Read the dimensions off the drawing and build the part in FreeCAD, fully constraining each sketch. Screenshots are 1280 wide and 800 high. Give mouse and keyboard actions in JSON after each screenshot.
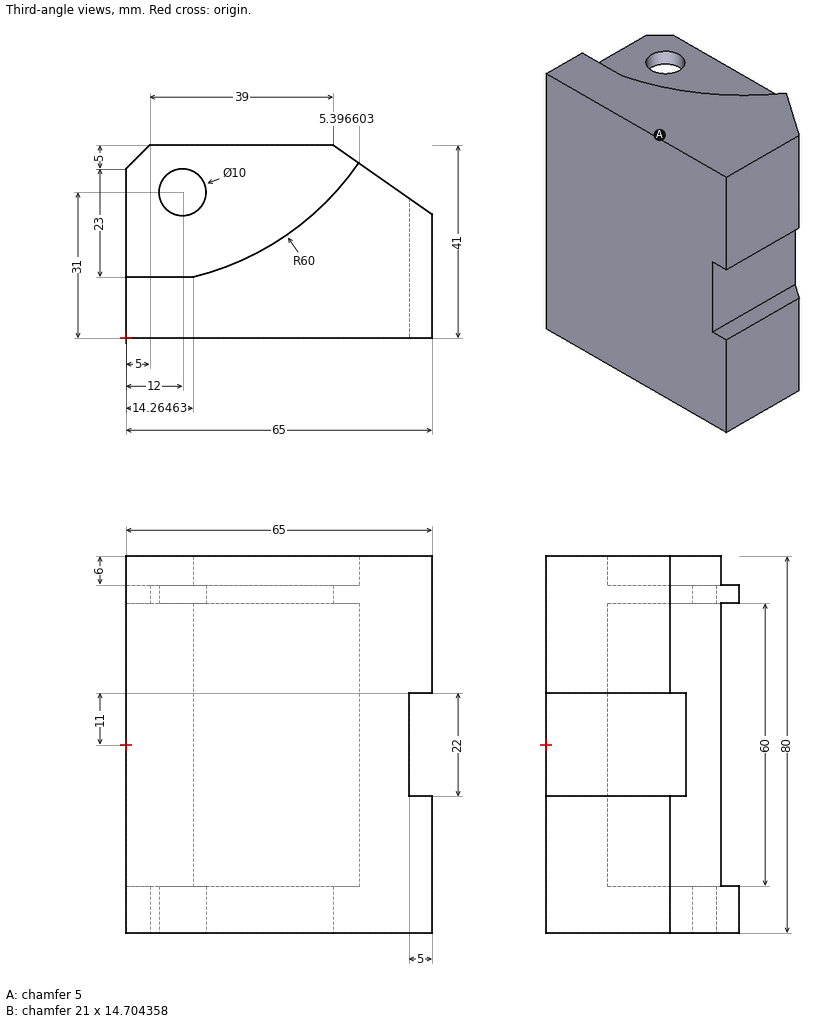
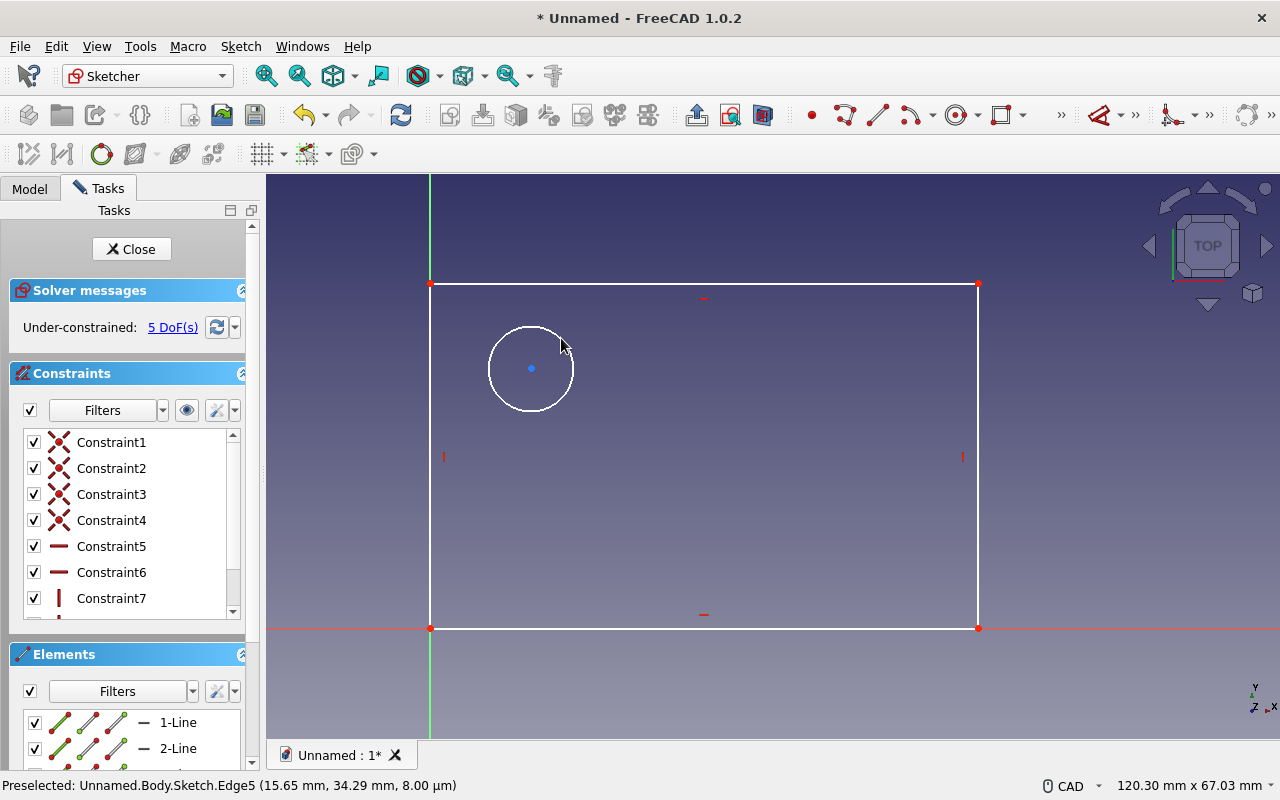
{"action": "key", "text": "d"}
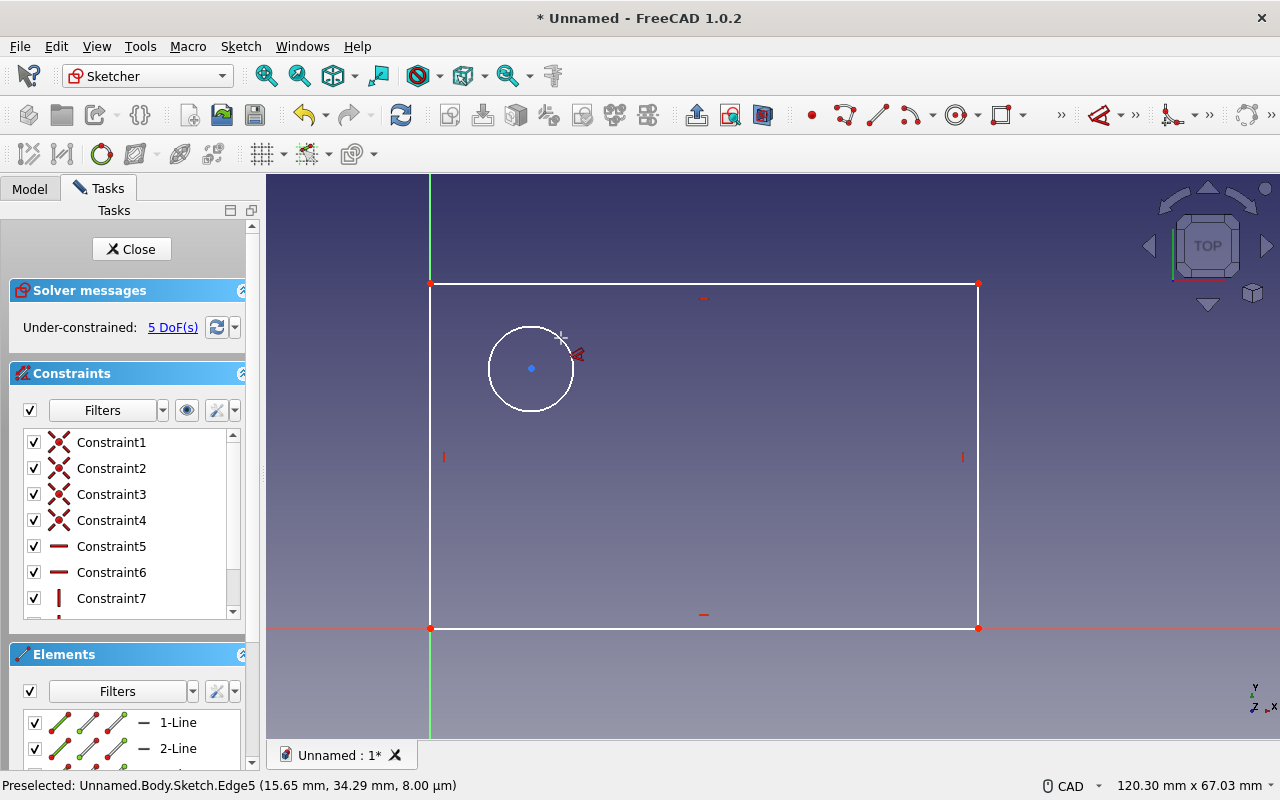
{"action": "left_click", "coordinate": [561, 339]}
{"action": "left_click", "coordinate": [584, 316]}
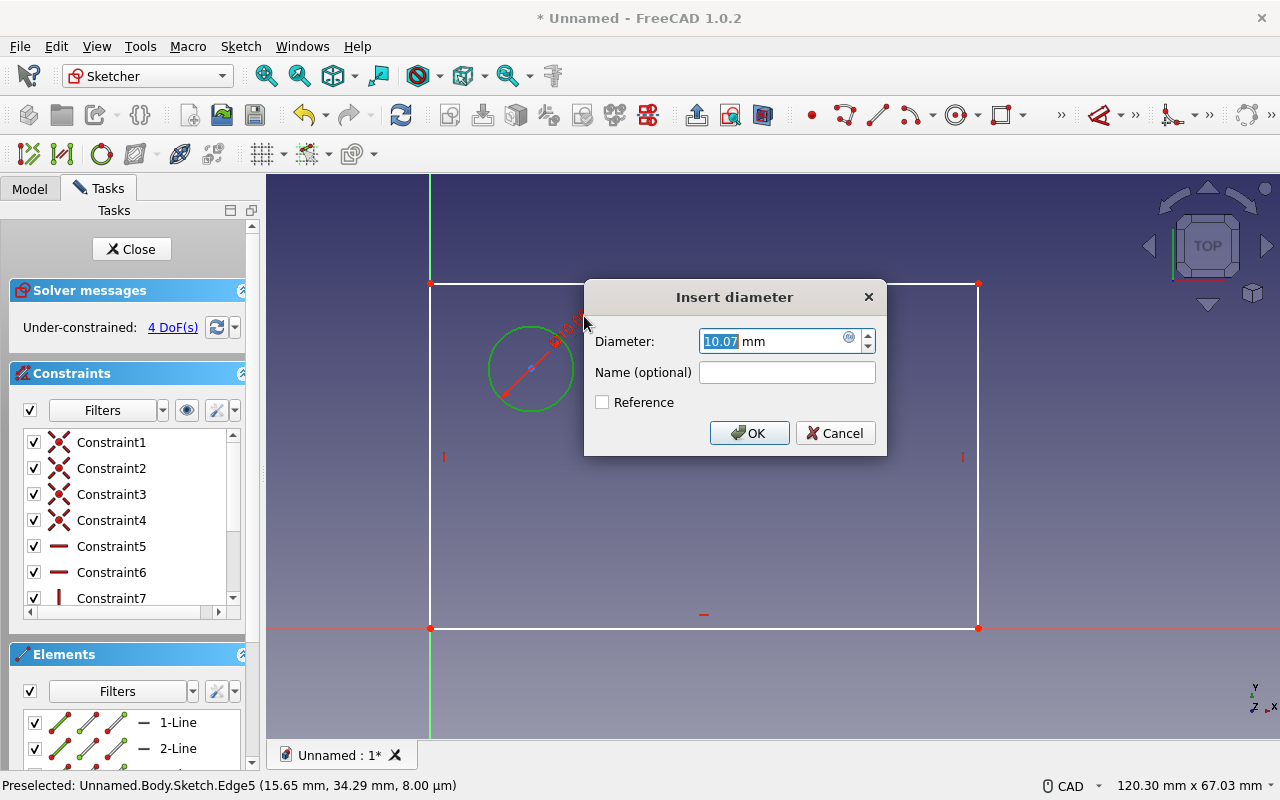
{"action": "type", "text": "10"}
{"action": "key", "text": "Return"}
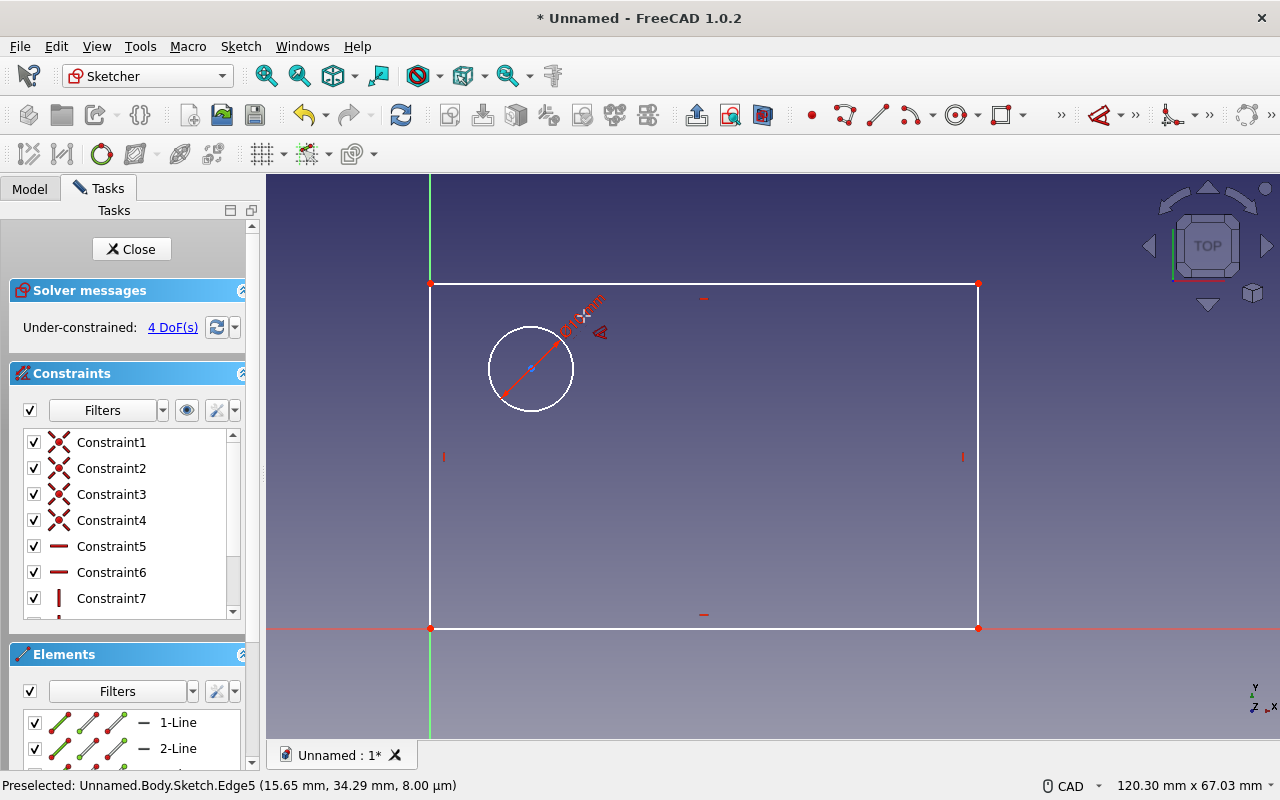
{"action": "left_click", "coordinate": [594, 629]}
{"action": "left_click", "coordinate": [704, 663]}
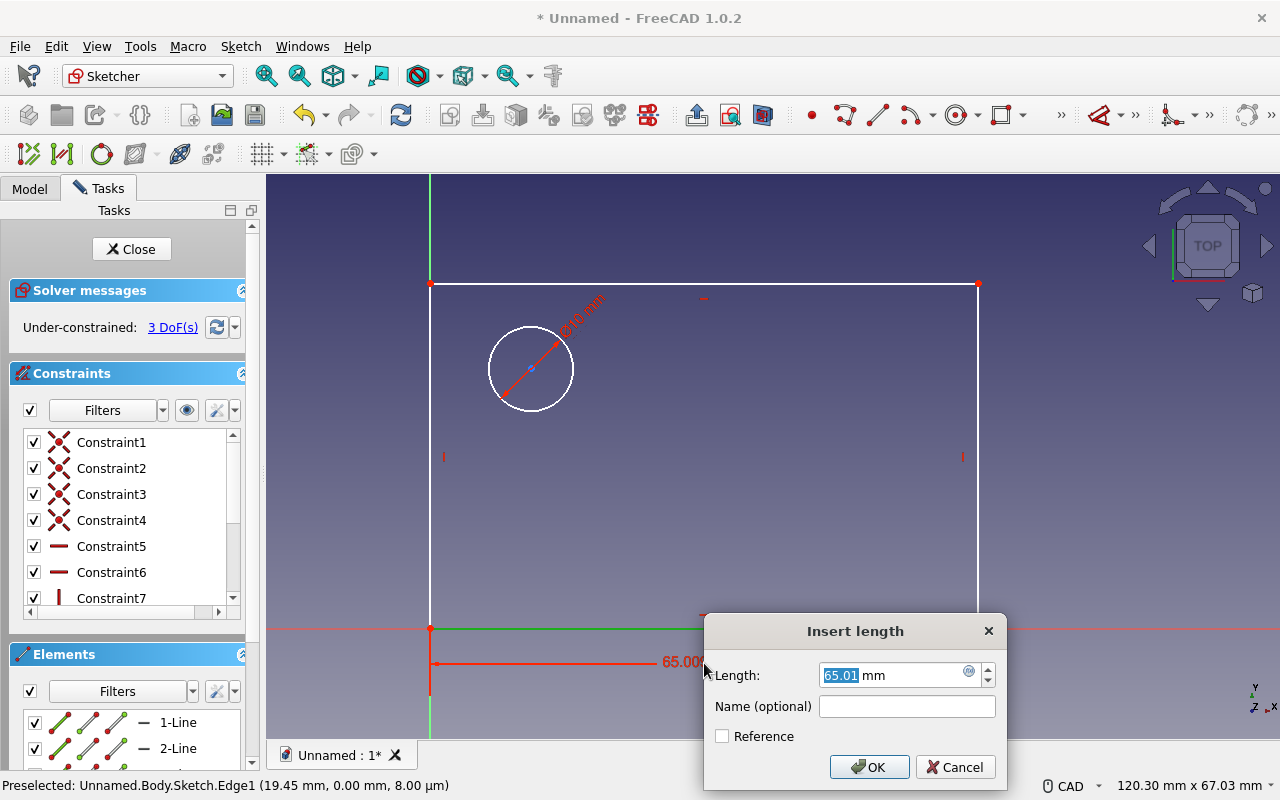
{"action": "type", "text": "65"}
{"action": "key", "text": "Return"}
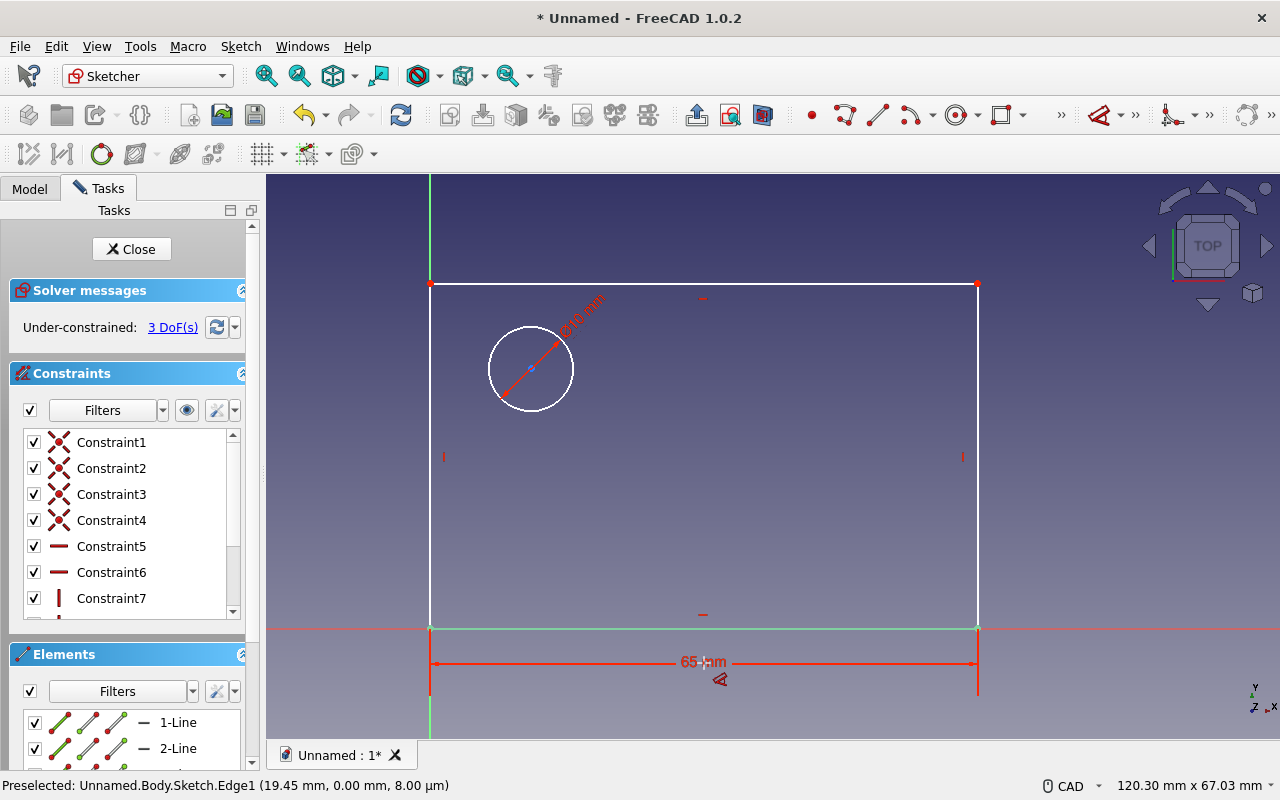
{"action": "left_click", "coordinate": [978, 525]}
{"action": "left_click", "coordinate": [1012, 456]}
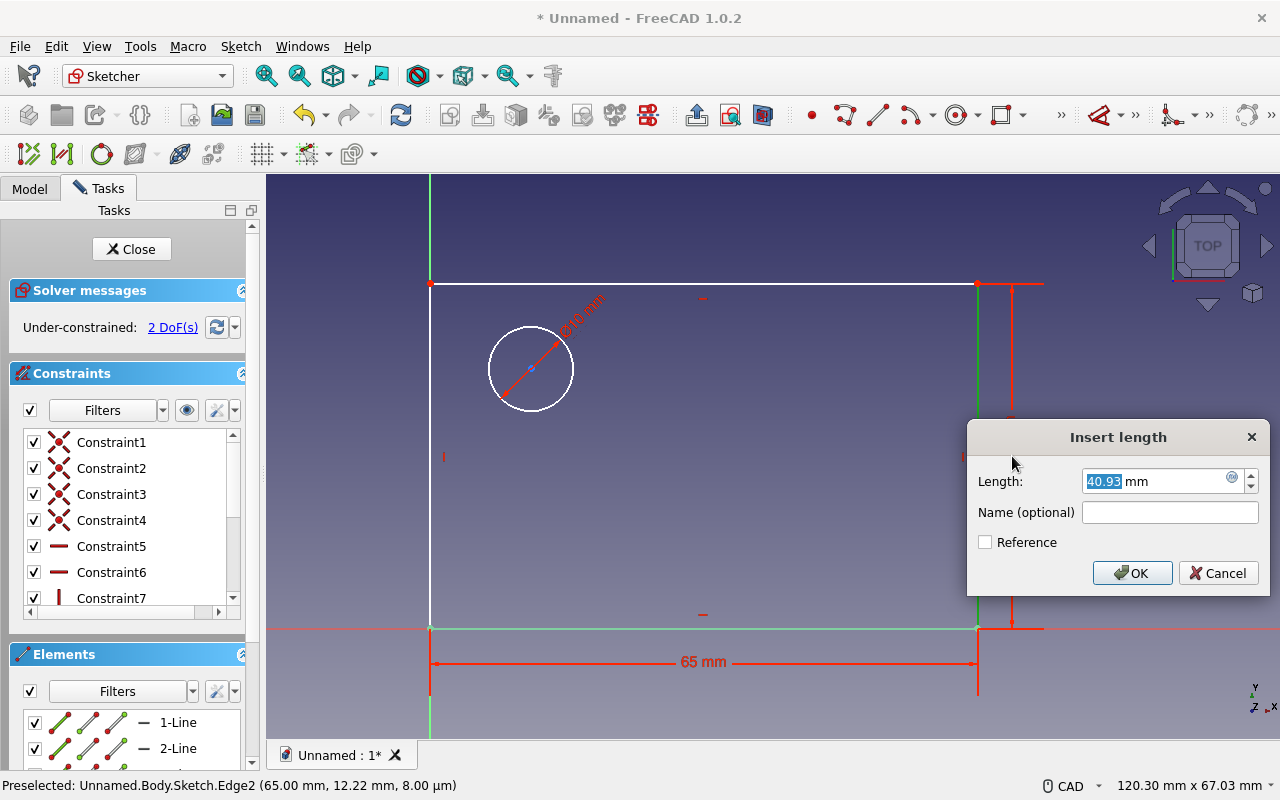
{"action": "type", "text": "41"}
{"action": "key", "text": "Return"}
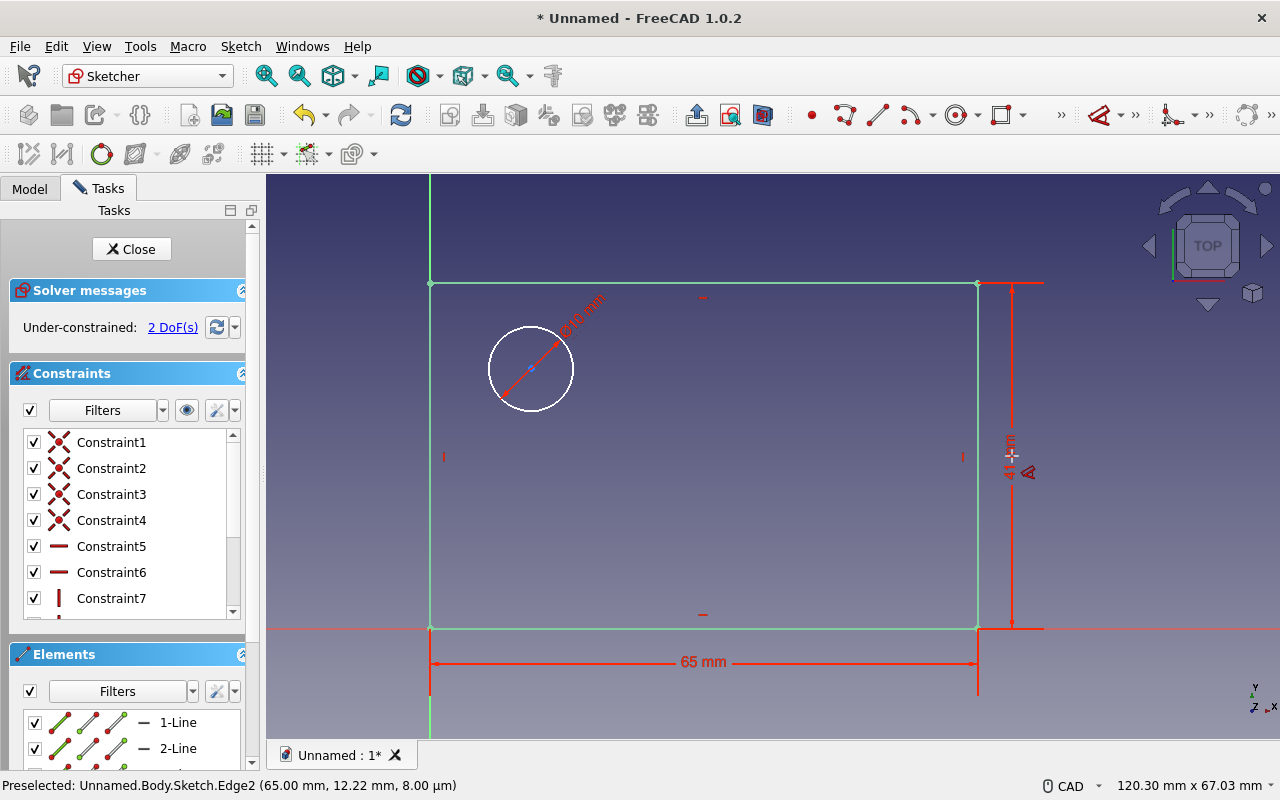
{"action": "left_click", "coordinate": [531, 369]}
{"action": "left_click", "coordinate": [481, 663]}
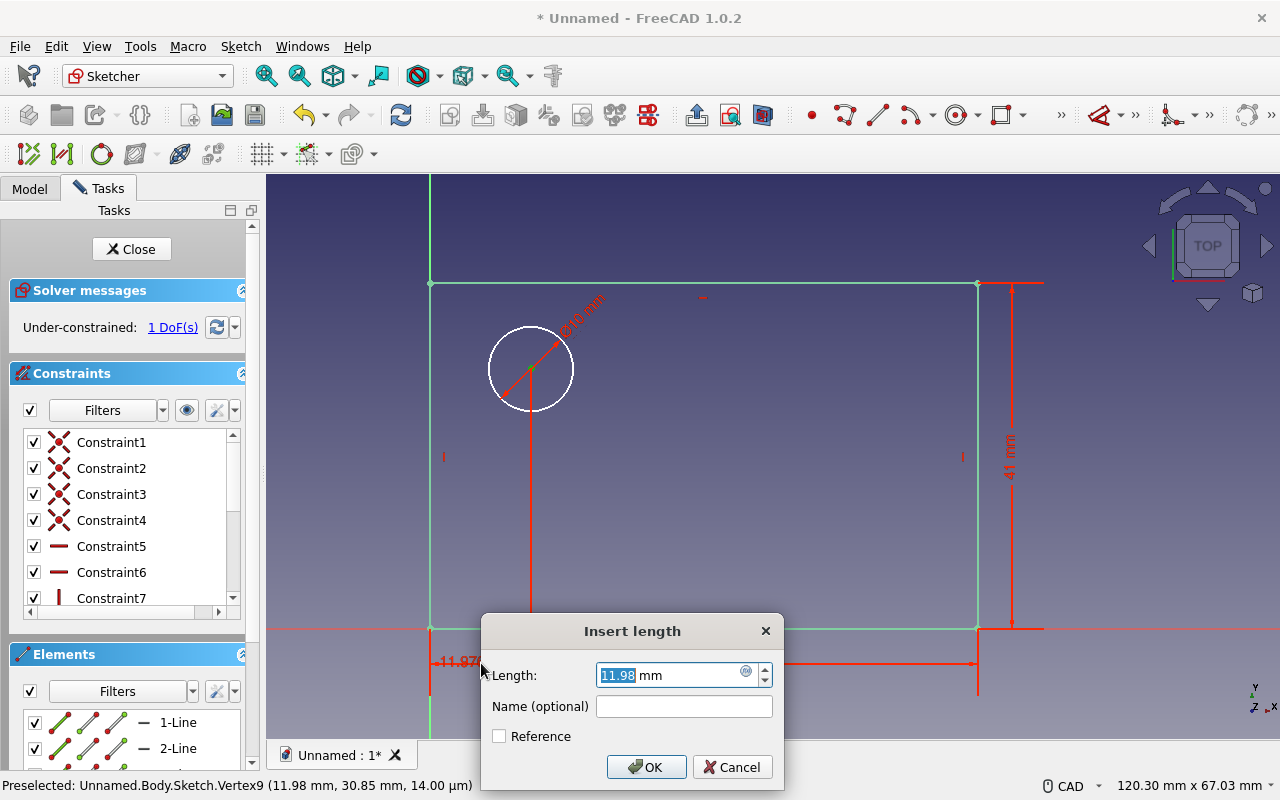
{"action": "type", "text": "12"}
{"action": "key", "text": "Return"}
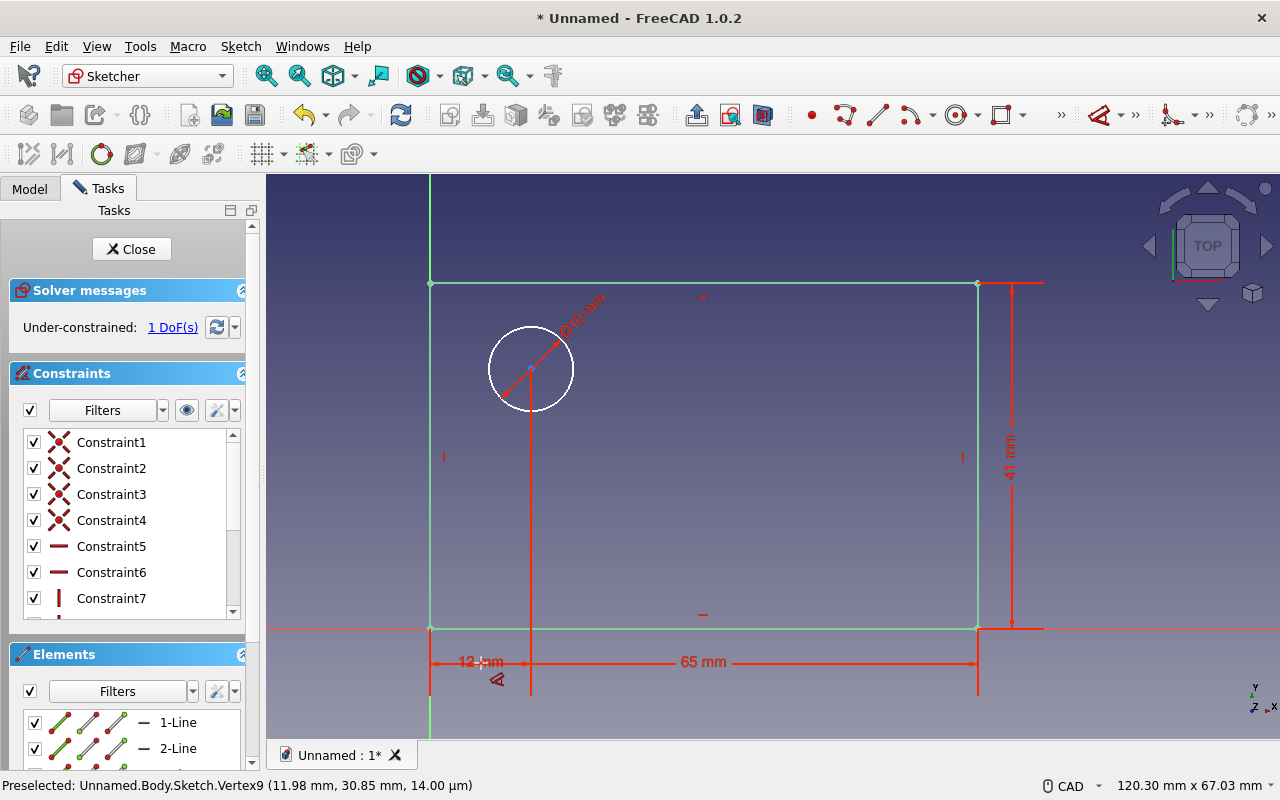
{"action": "left_click", "coordinate": [531, 369]}
{"action": "left_click", "coordinate": [396, 499]}